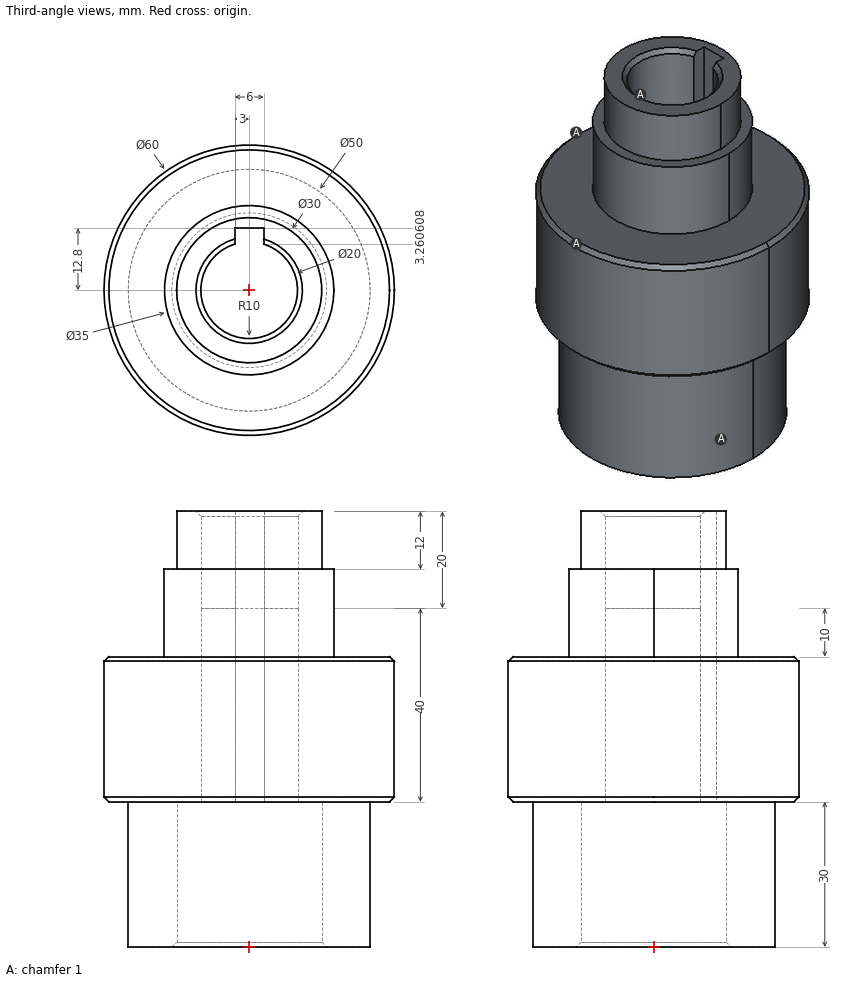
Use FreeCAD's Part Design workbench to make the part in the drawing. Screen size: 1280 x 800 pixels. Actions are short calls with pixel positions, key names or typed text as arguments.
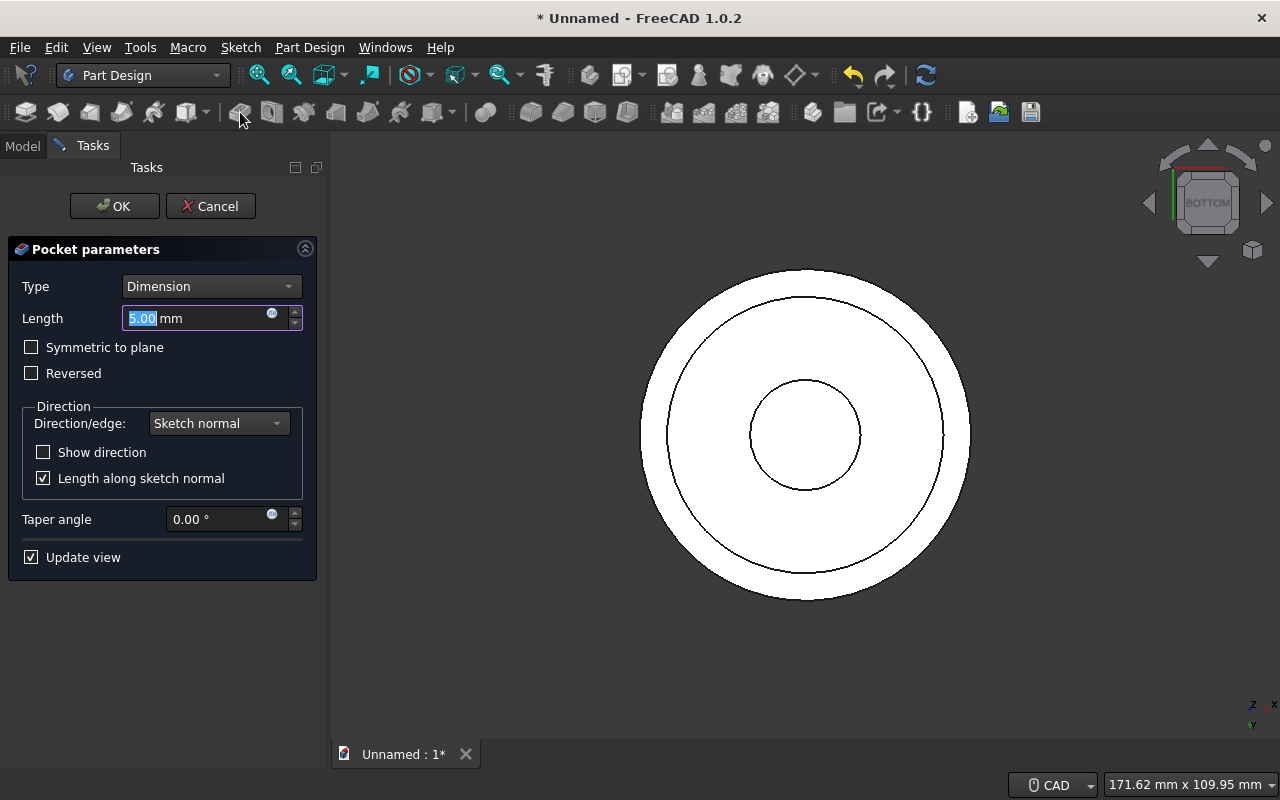
click(212, 286)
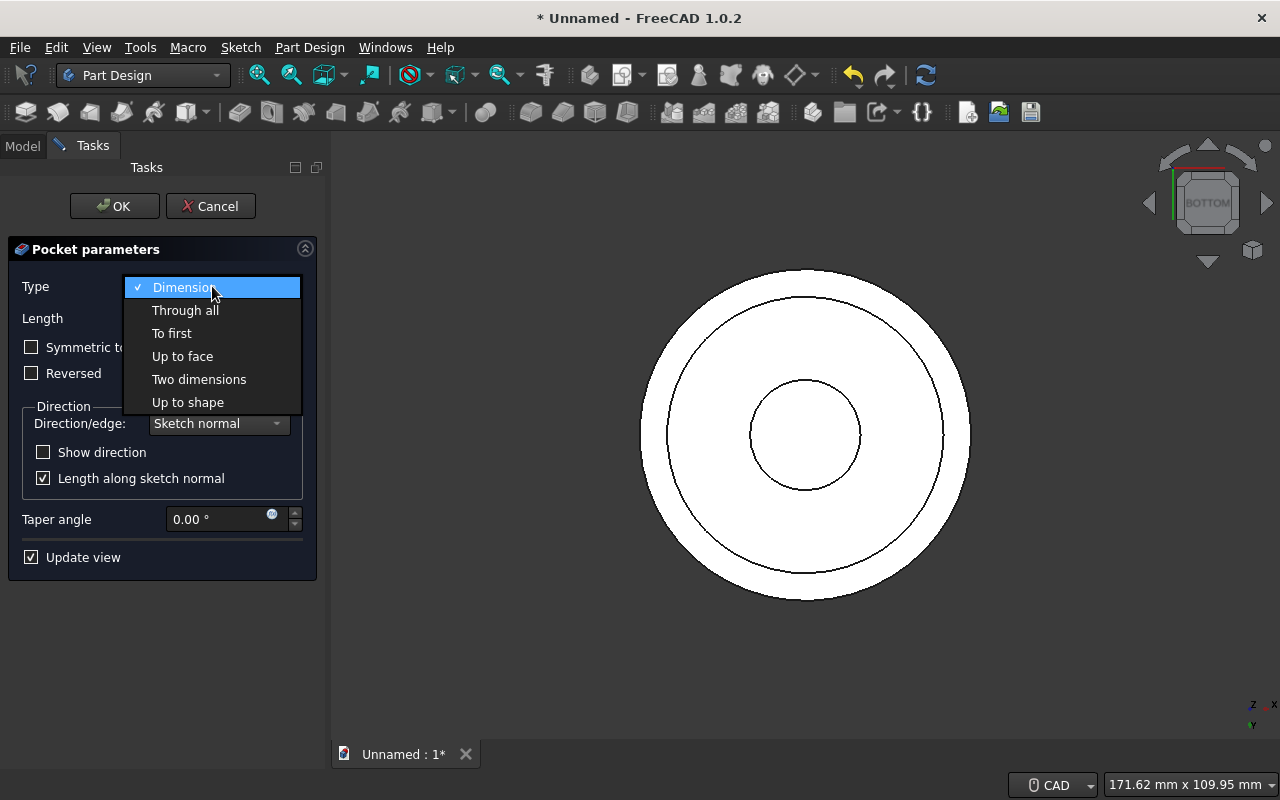
click(212, 310)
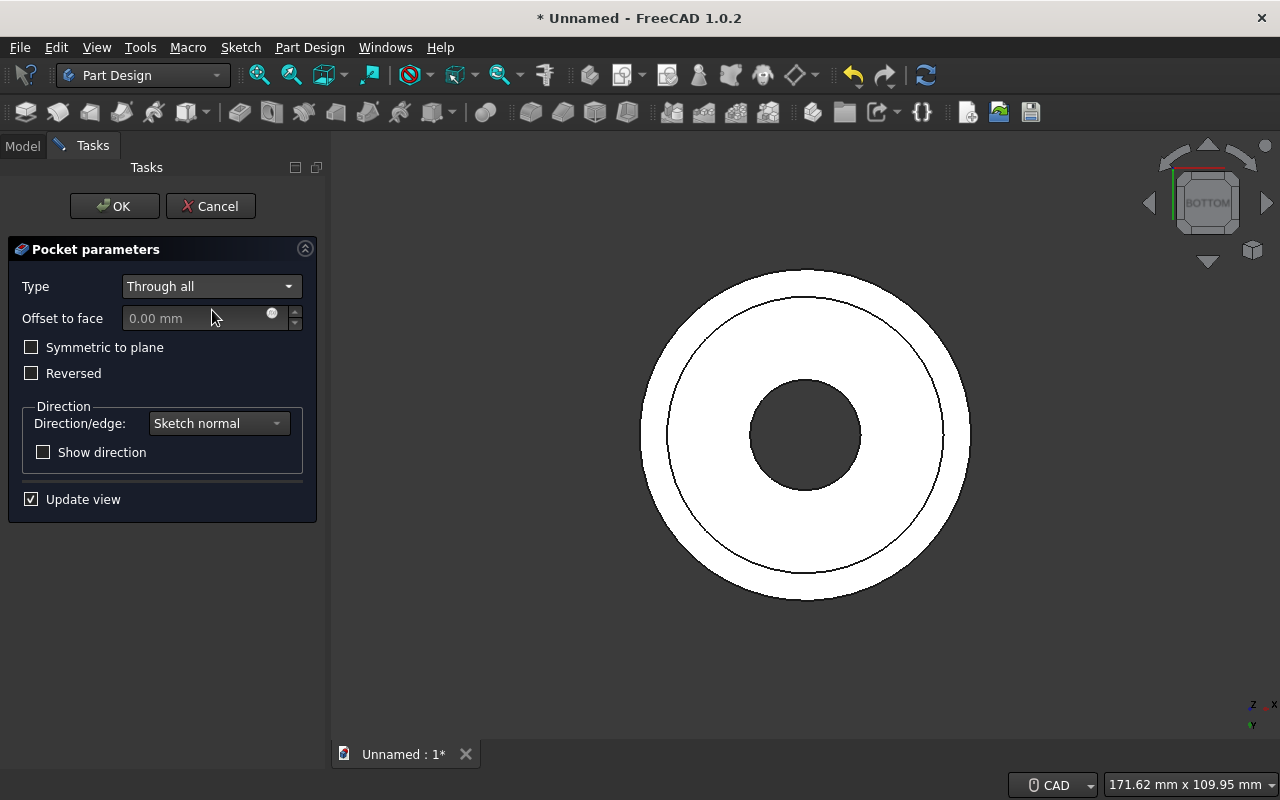
click(115, 206)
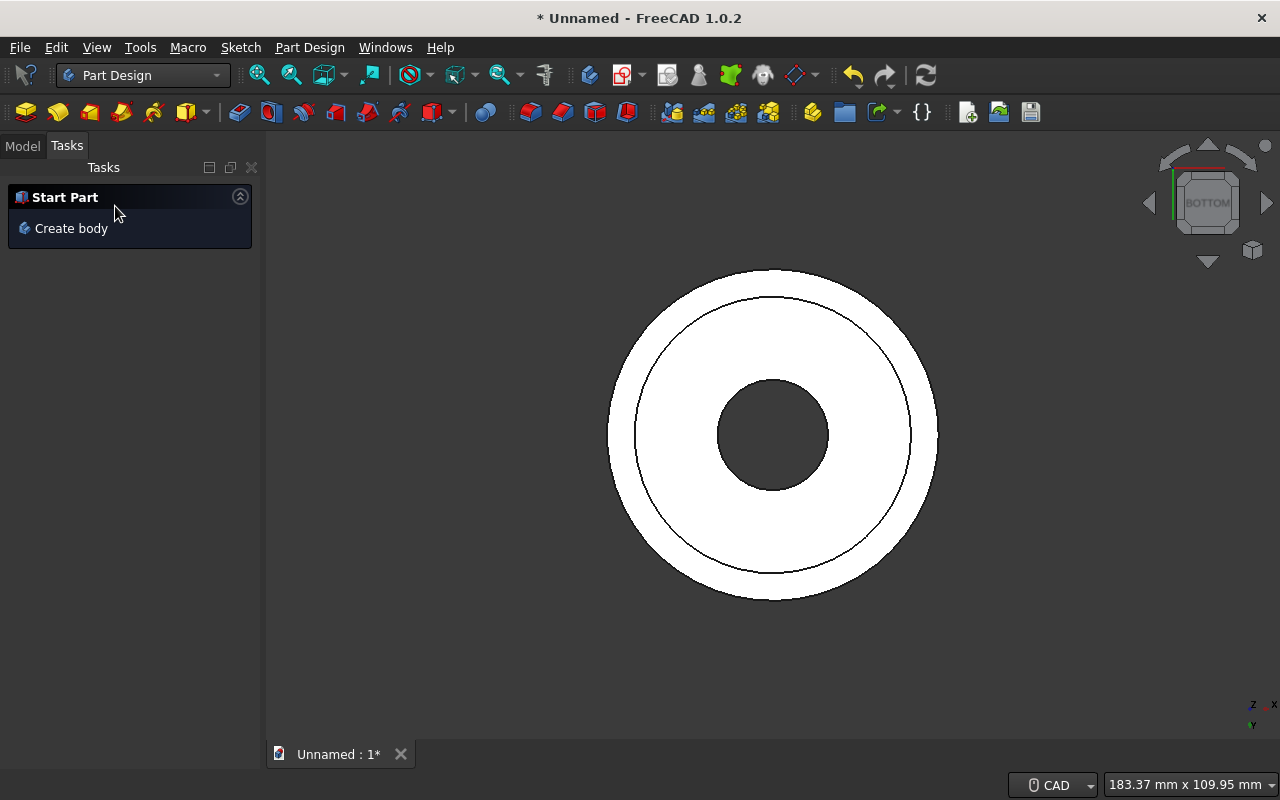
key(0)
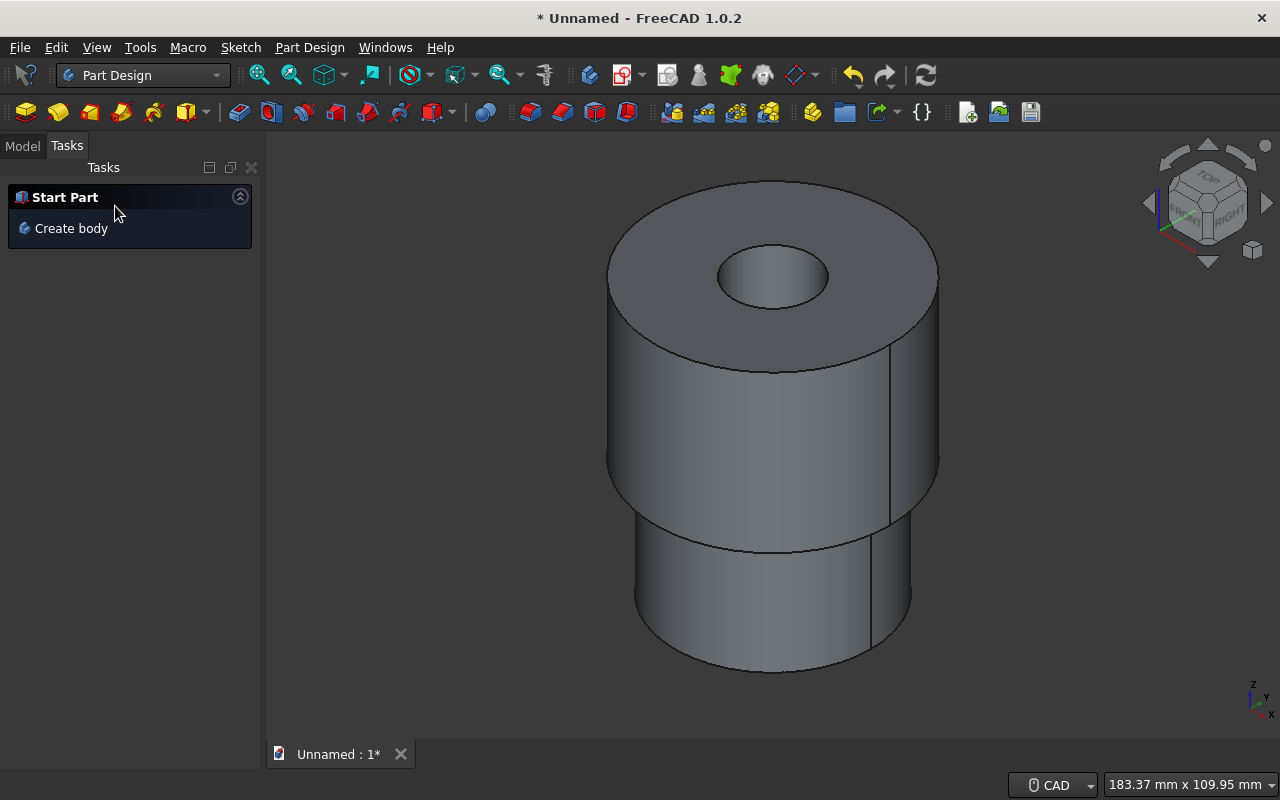
click(806, 218)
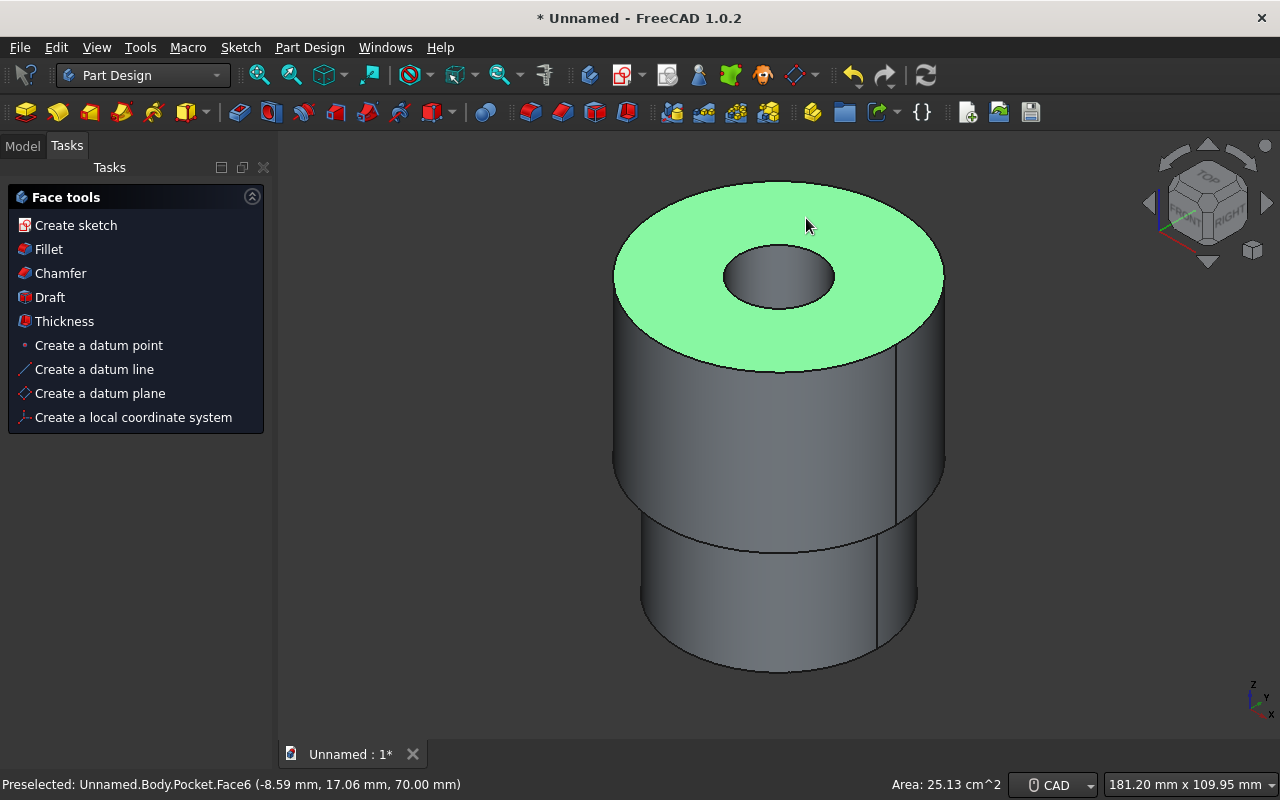
click(622, 76)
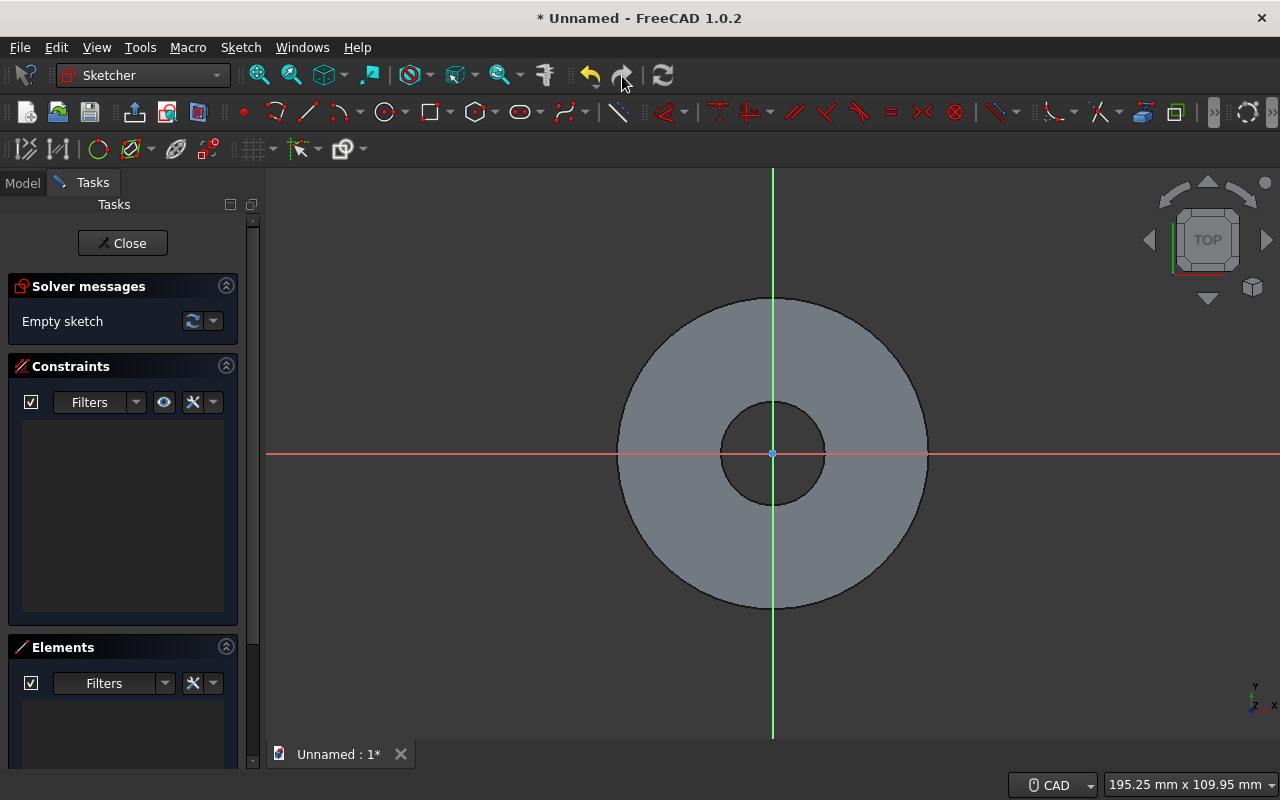
scroll(790, 412, up, 8)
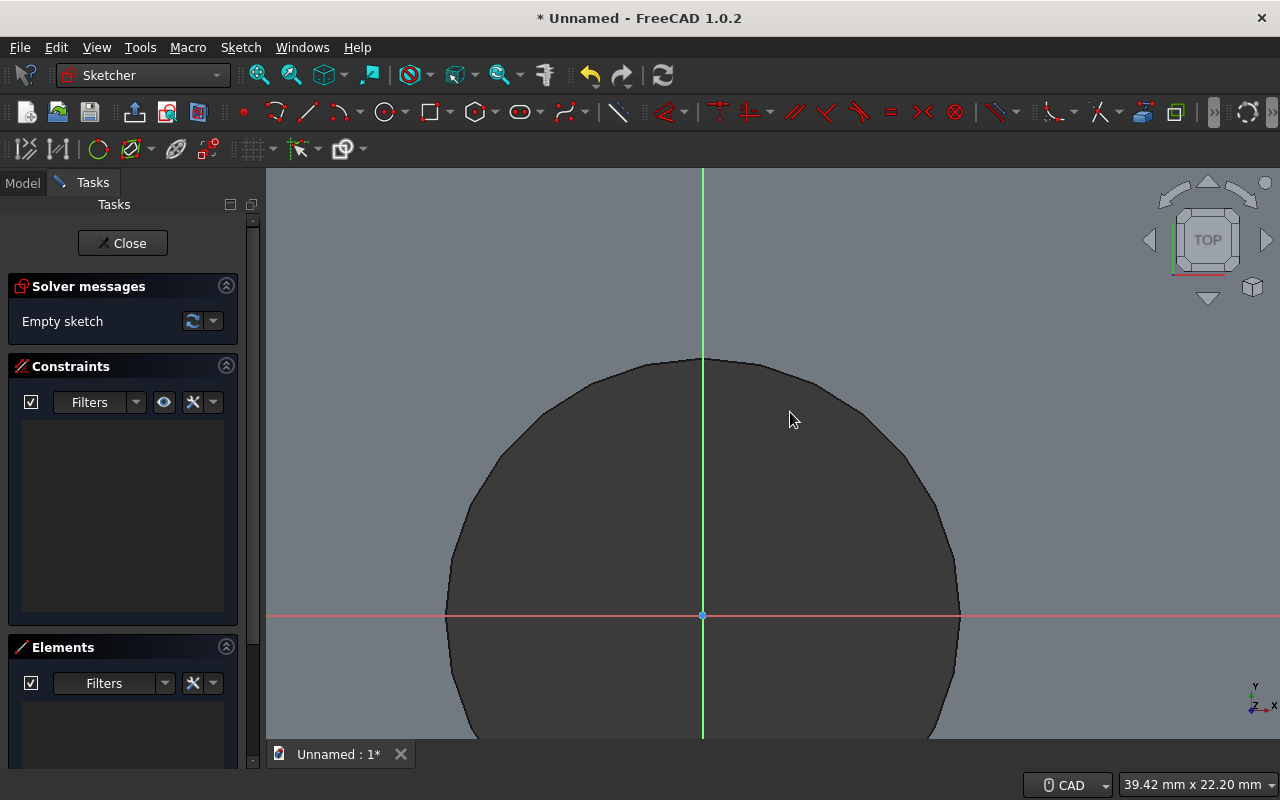
click(430, 112)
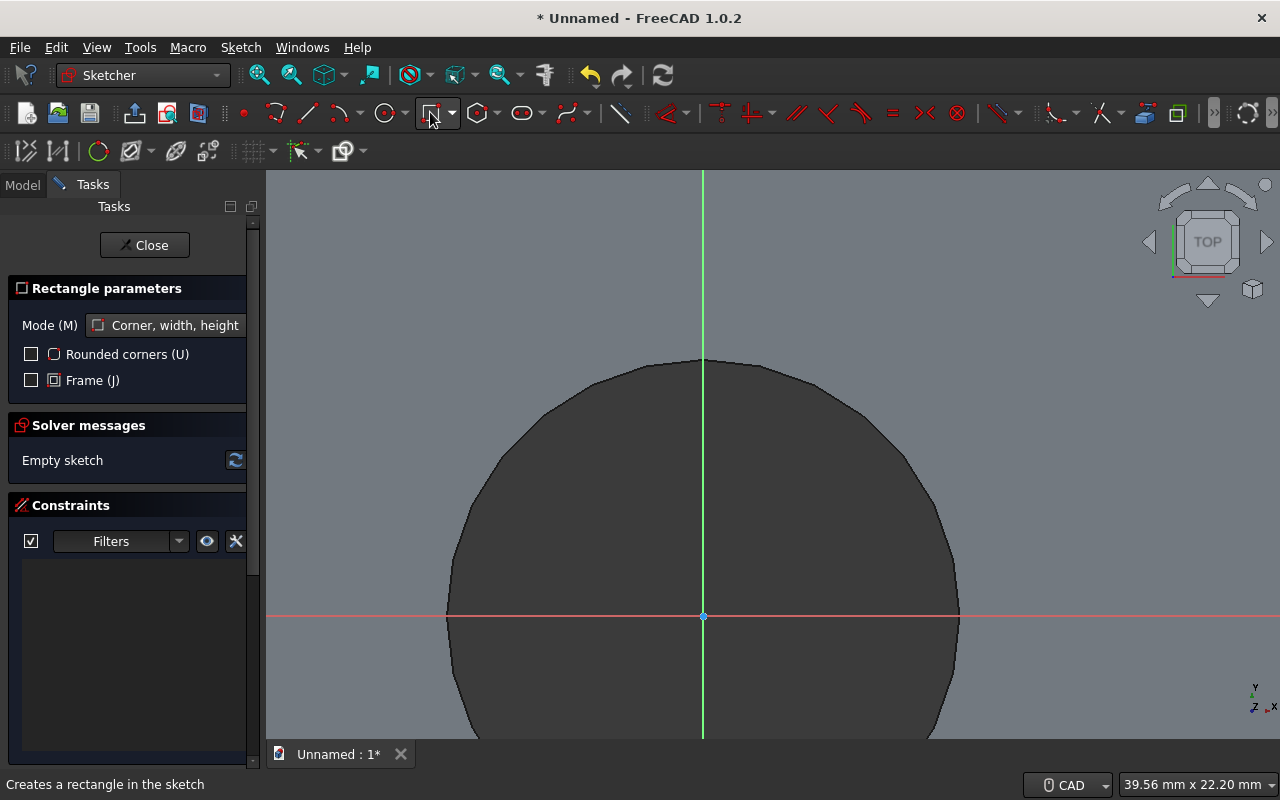
click(626, 288)
move(780, 372)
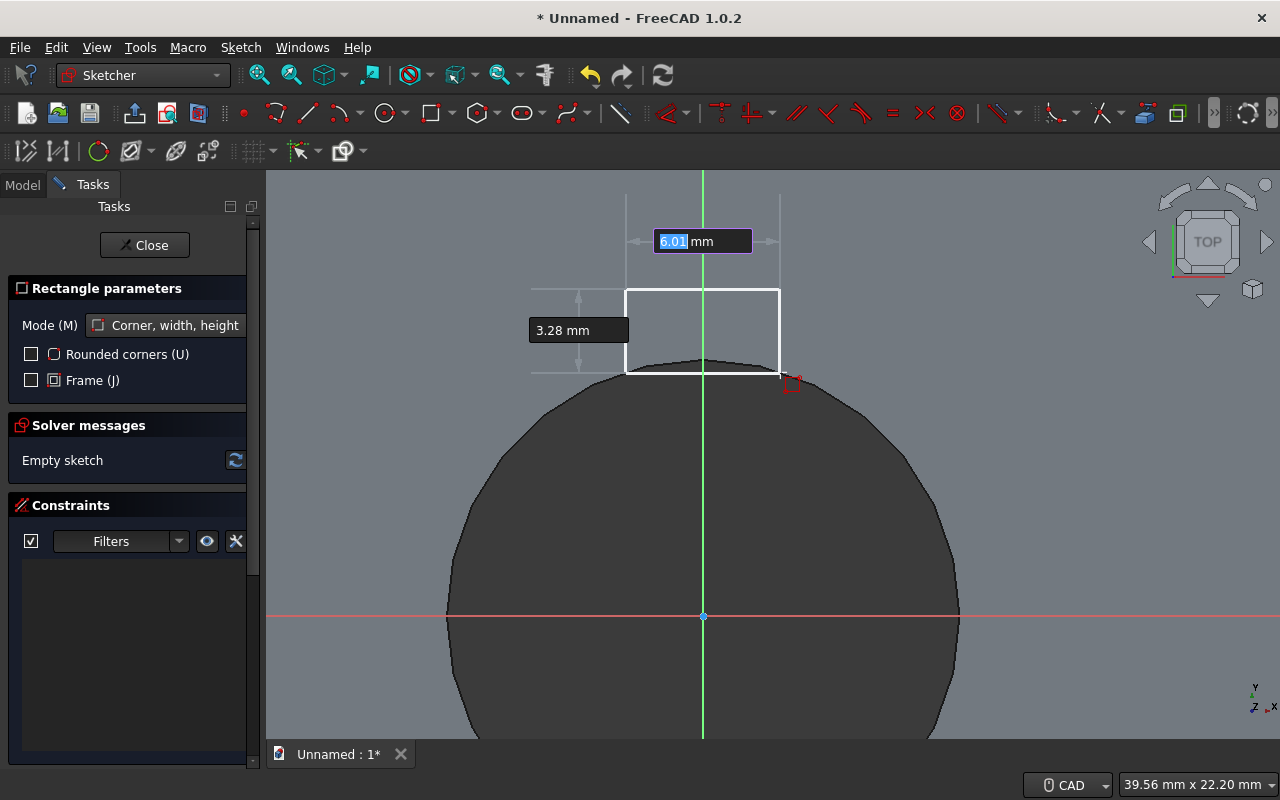
text(6)
key(Tab)
text(3.260608)
key(Return)
key(Escape)